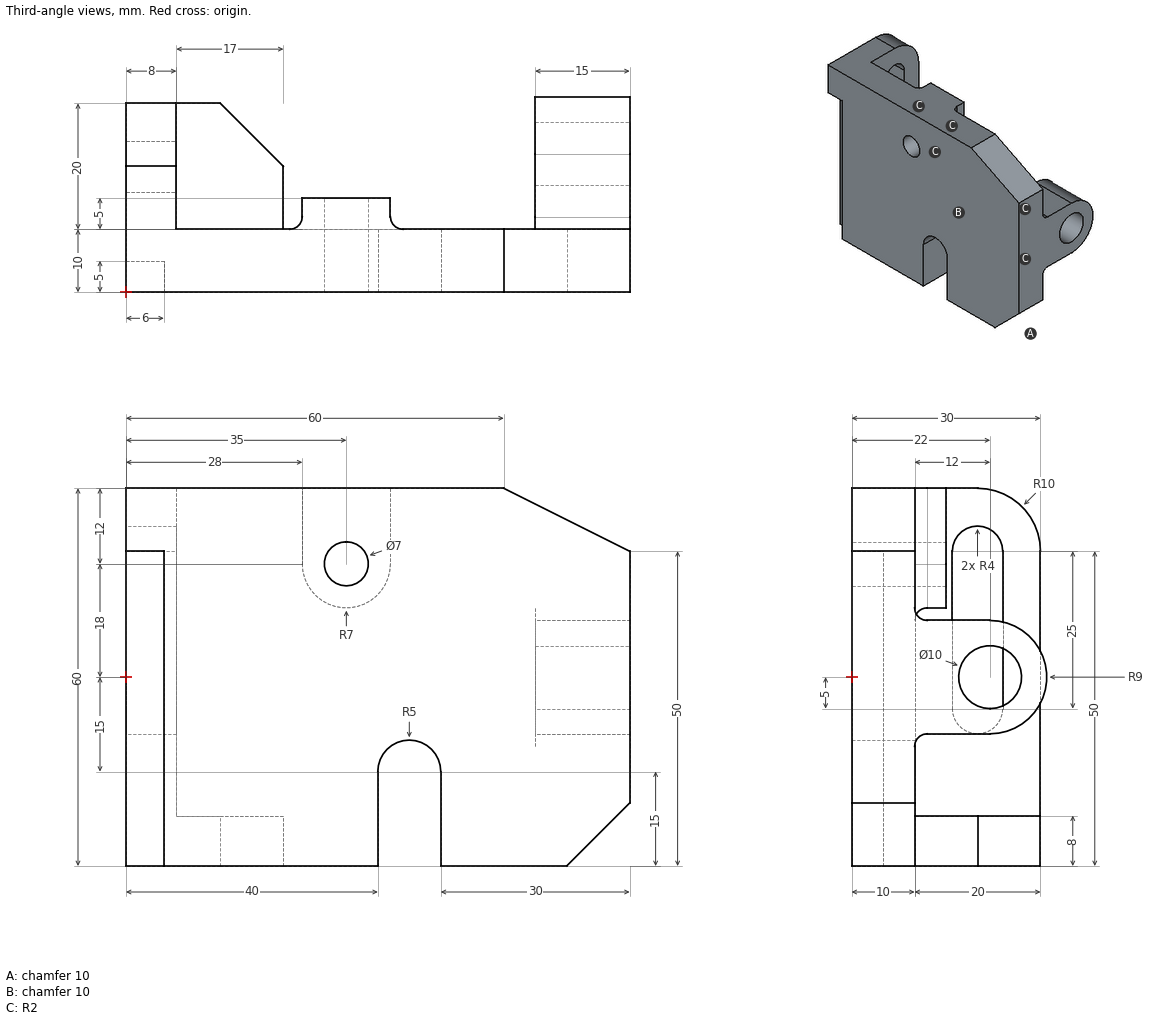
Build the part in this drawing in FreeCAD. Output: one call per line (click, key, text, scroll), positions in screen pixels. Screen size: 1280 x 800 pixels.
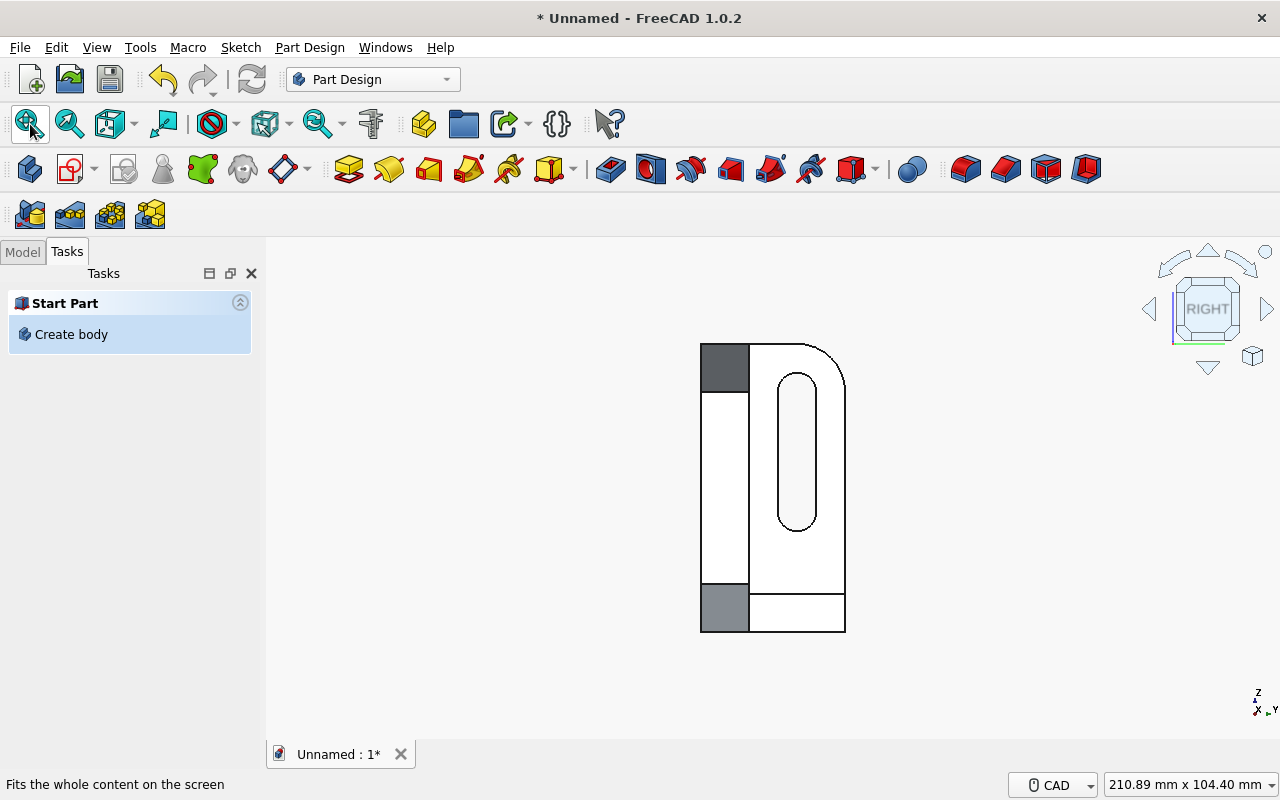
click(845, 612)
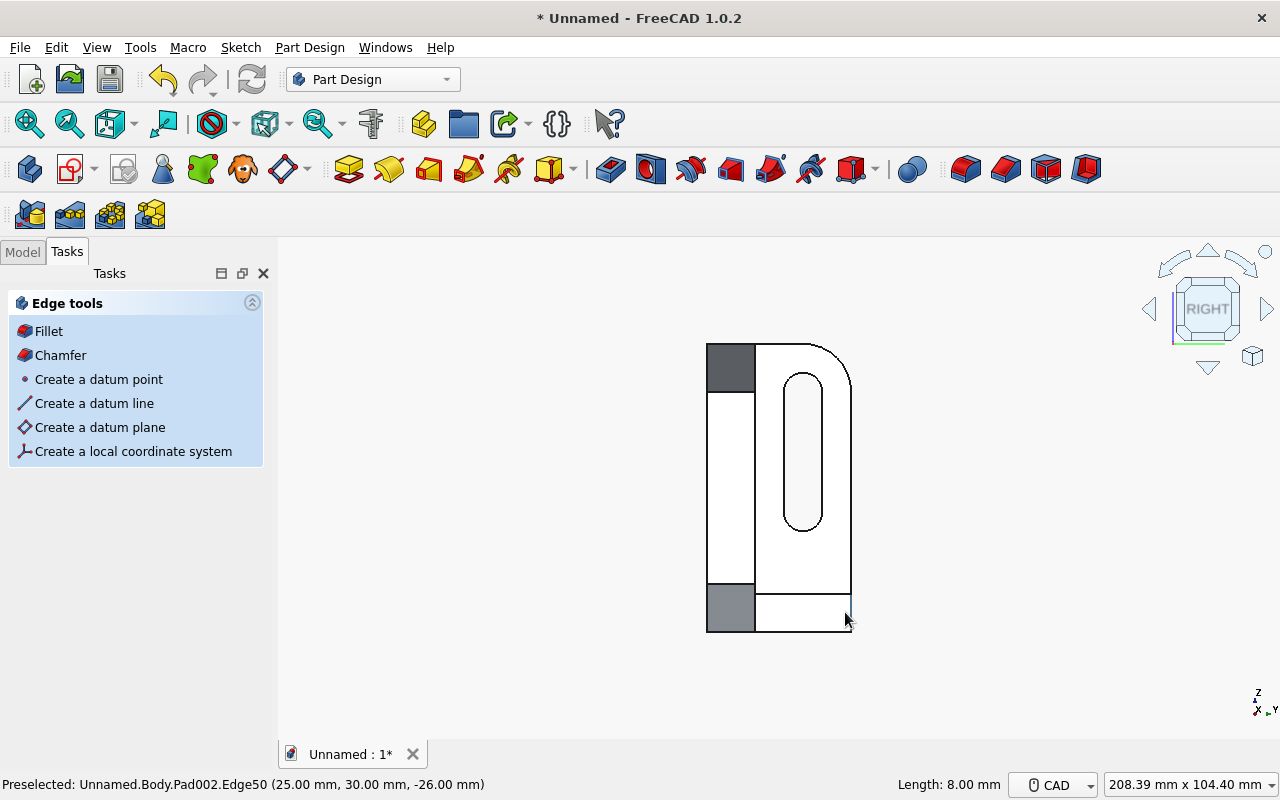
click(1006, 170)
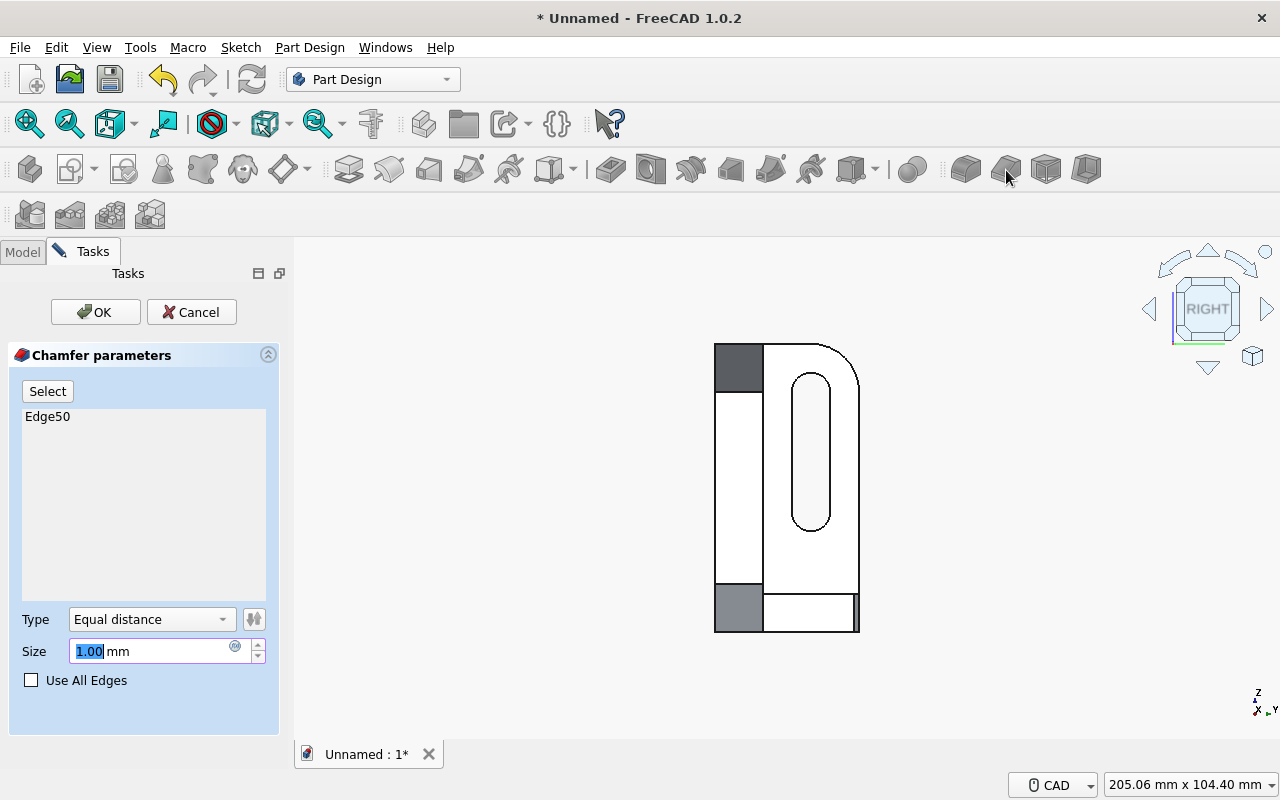
text(10)
key(Tab)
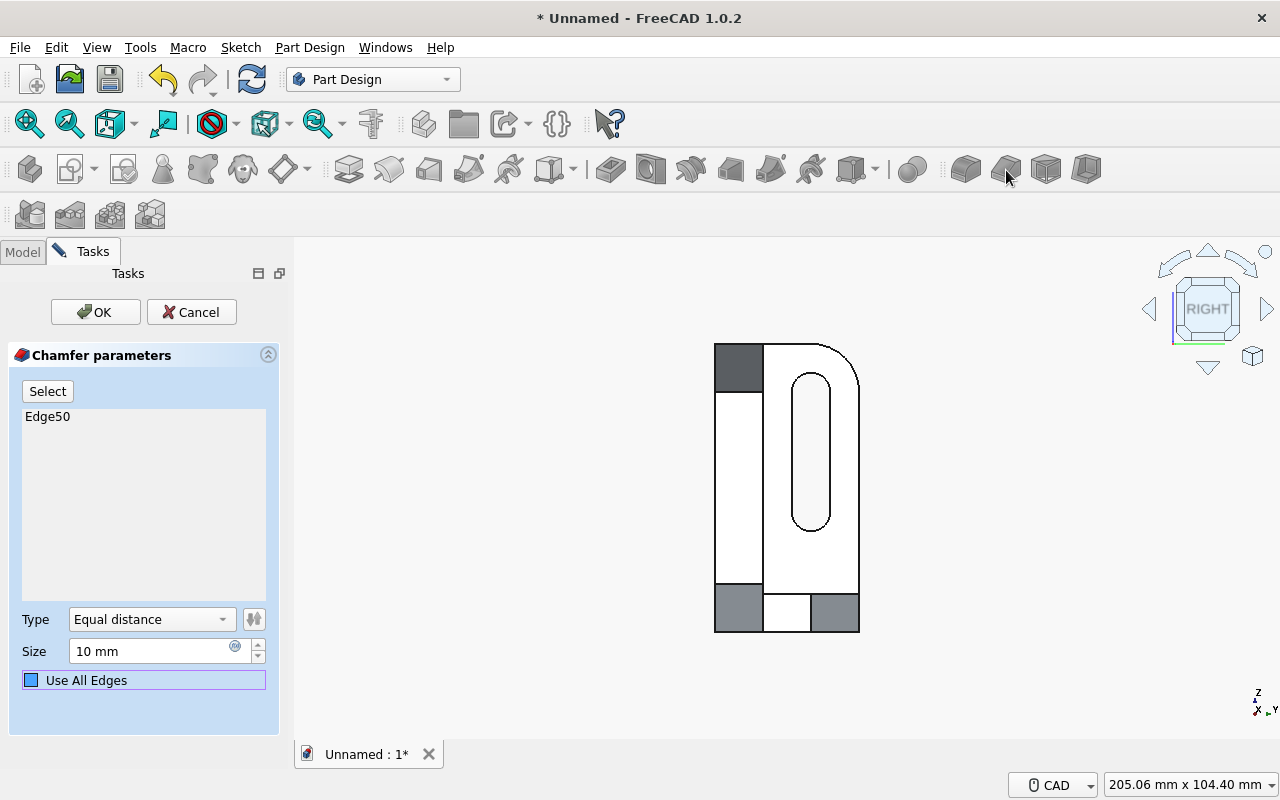
click(96, 312)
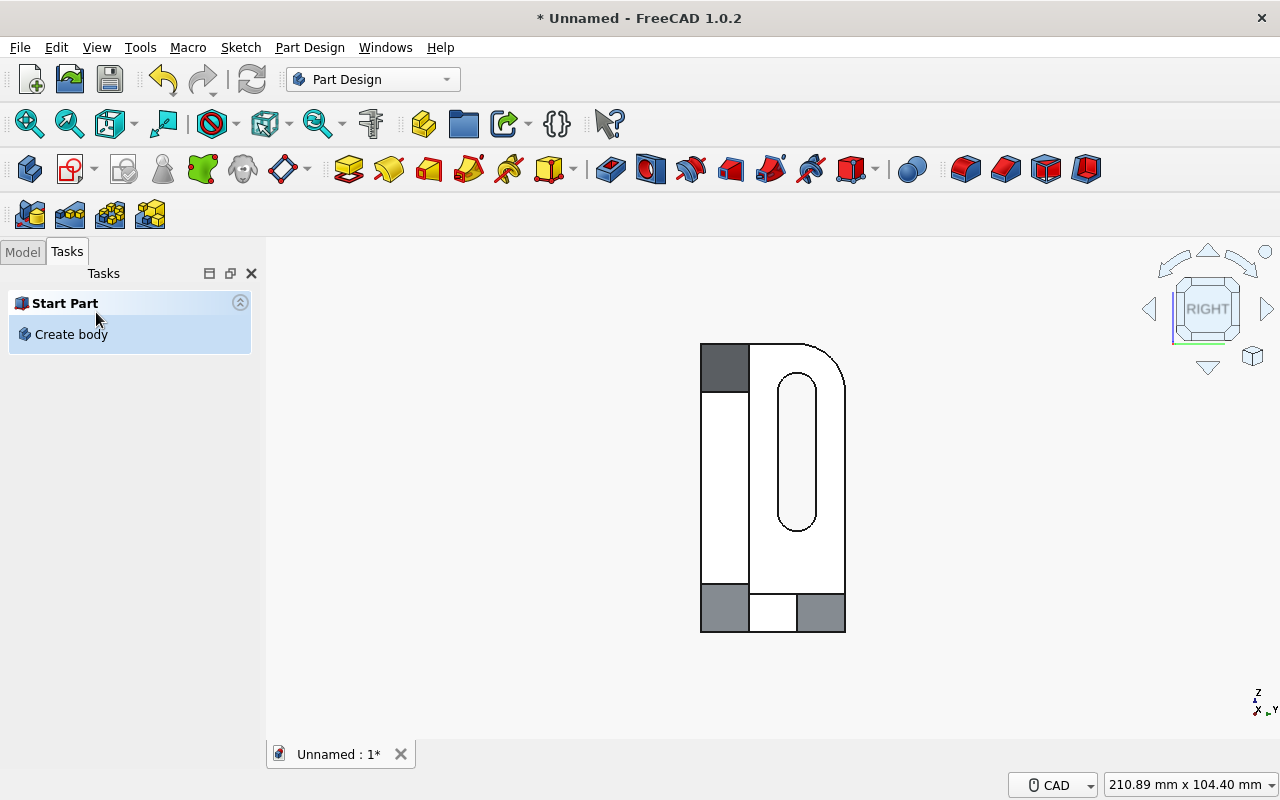
key(4)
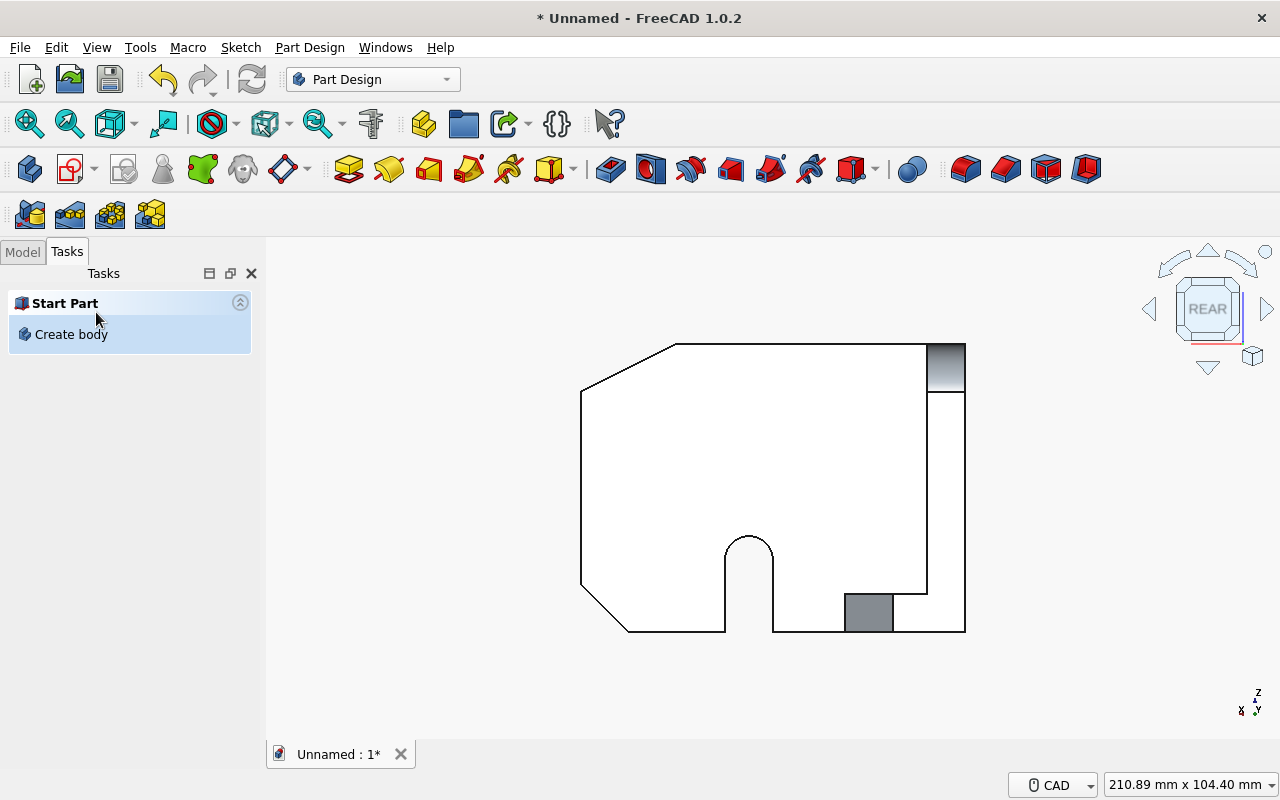
click(803, 446)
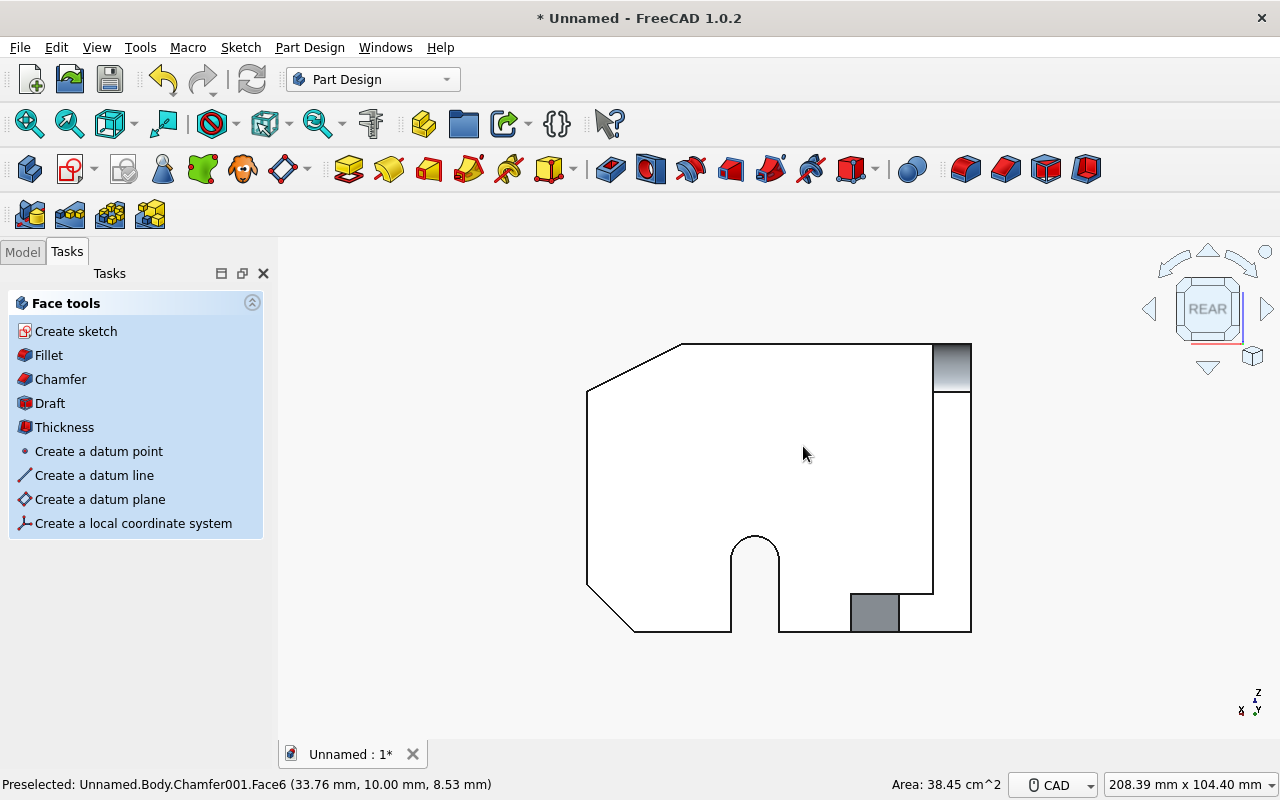
click(70, 170)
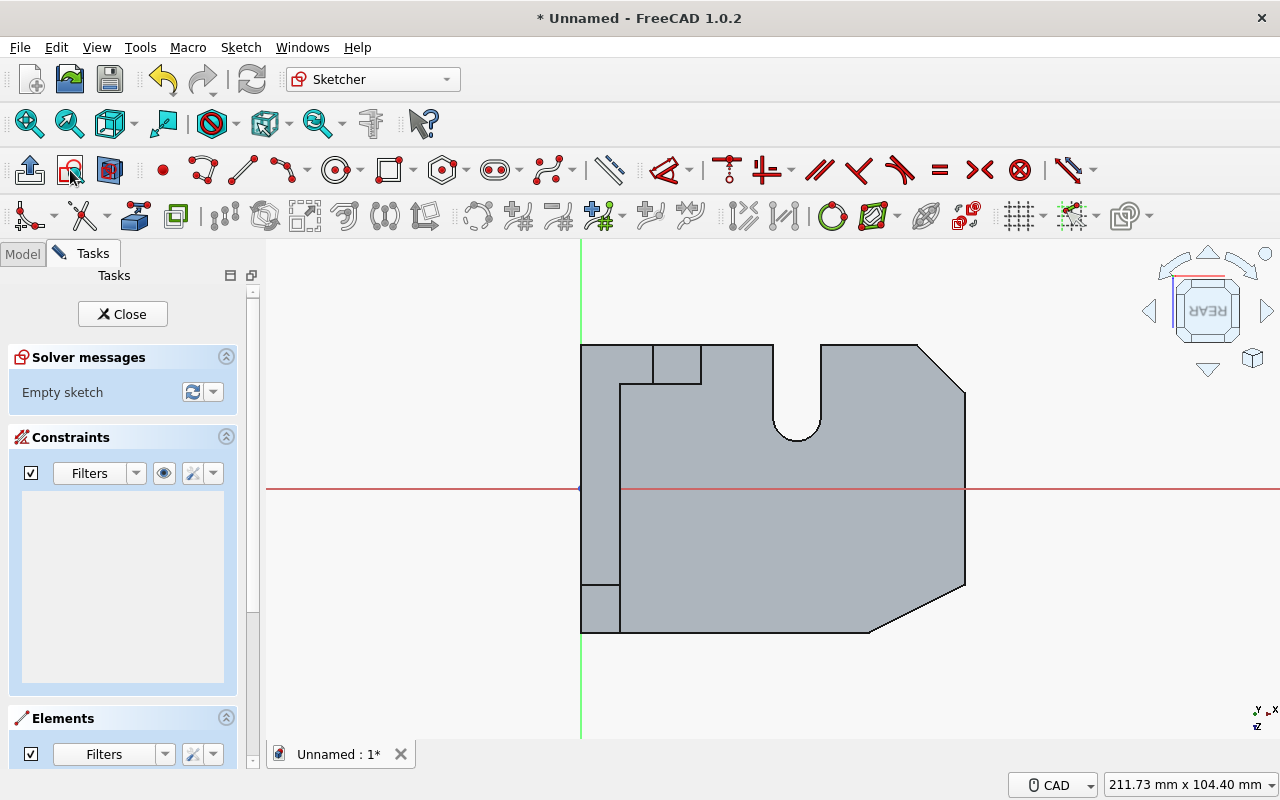
click(110, 170)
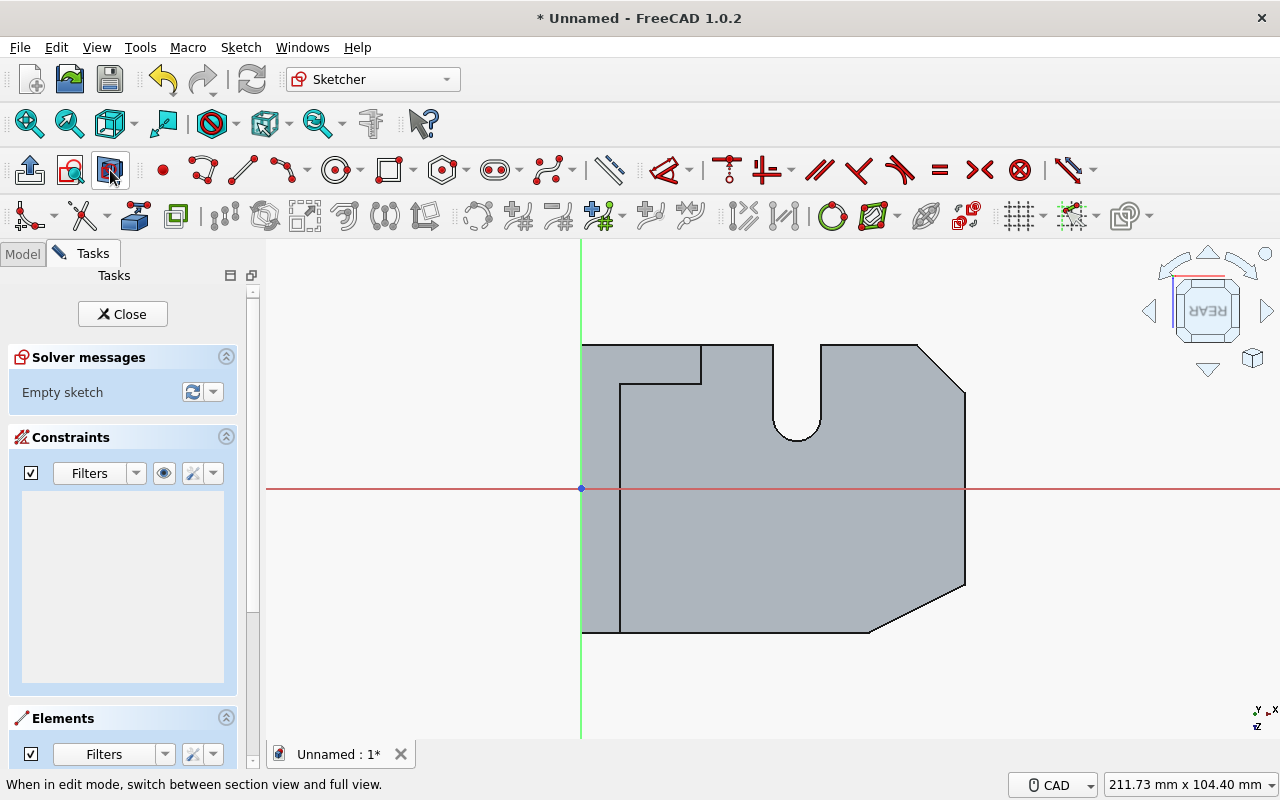
scroll(664, 619, up, 4)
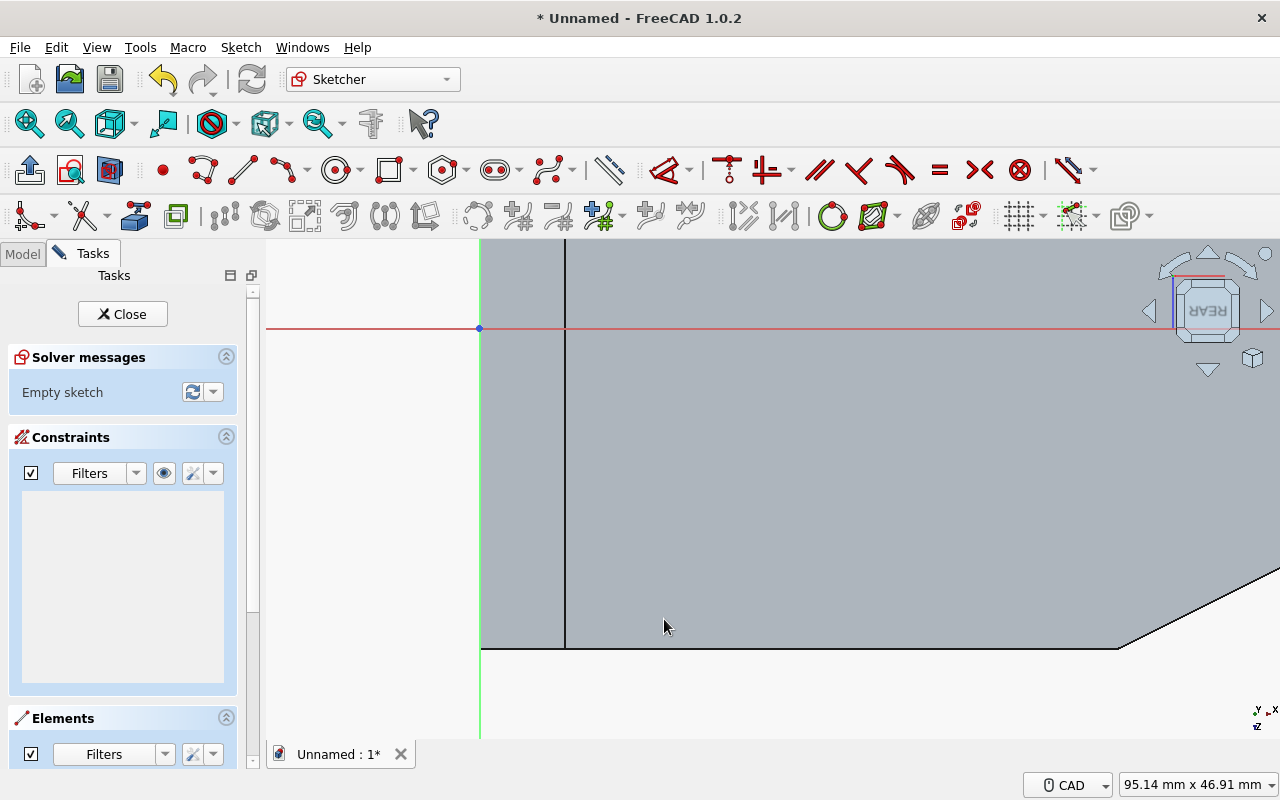
click(204, 170)